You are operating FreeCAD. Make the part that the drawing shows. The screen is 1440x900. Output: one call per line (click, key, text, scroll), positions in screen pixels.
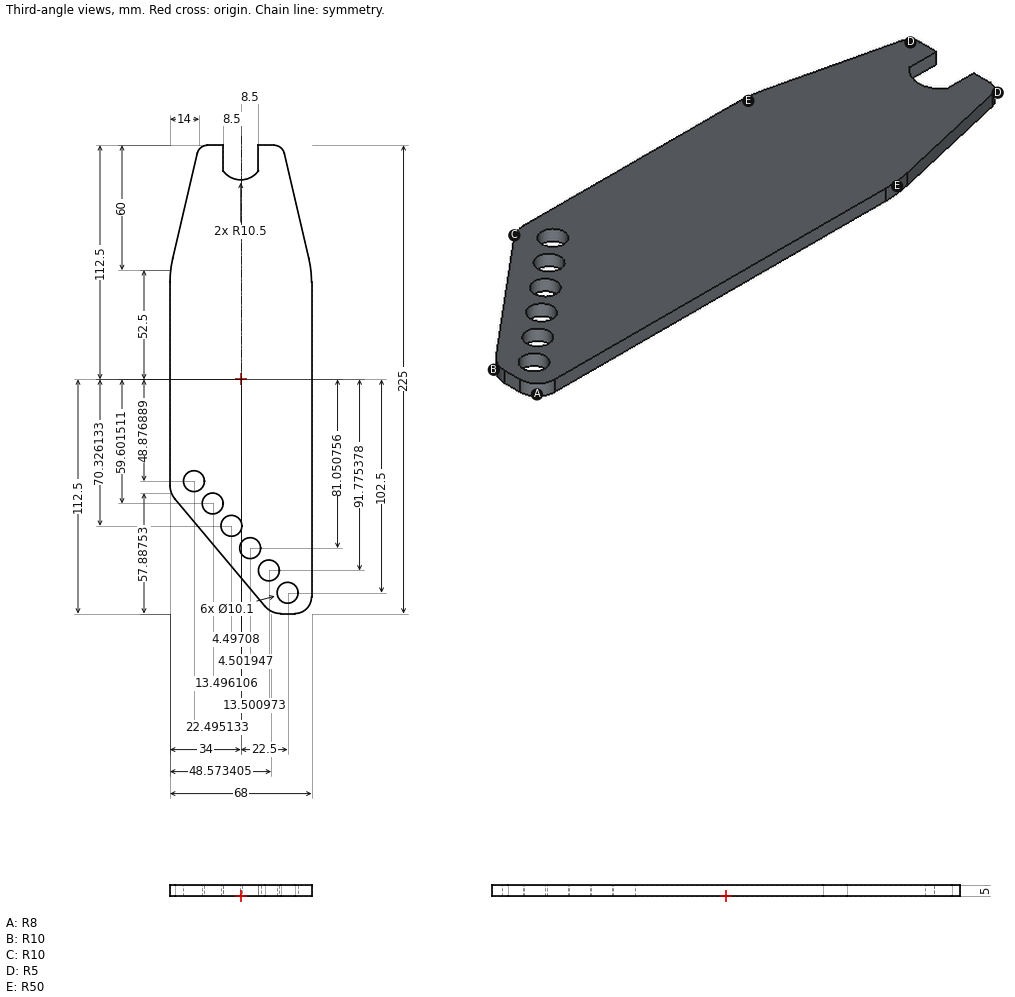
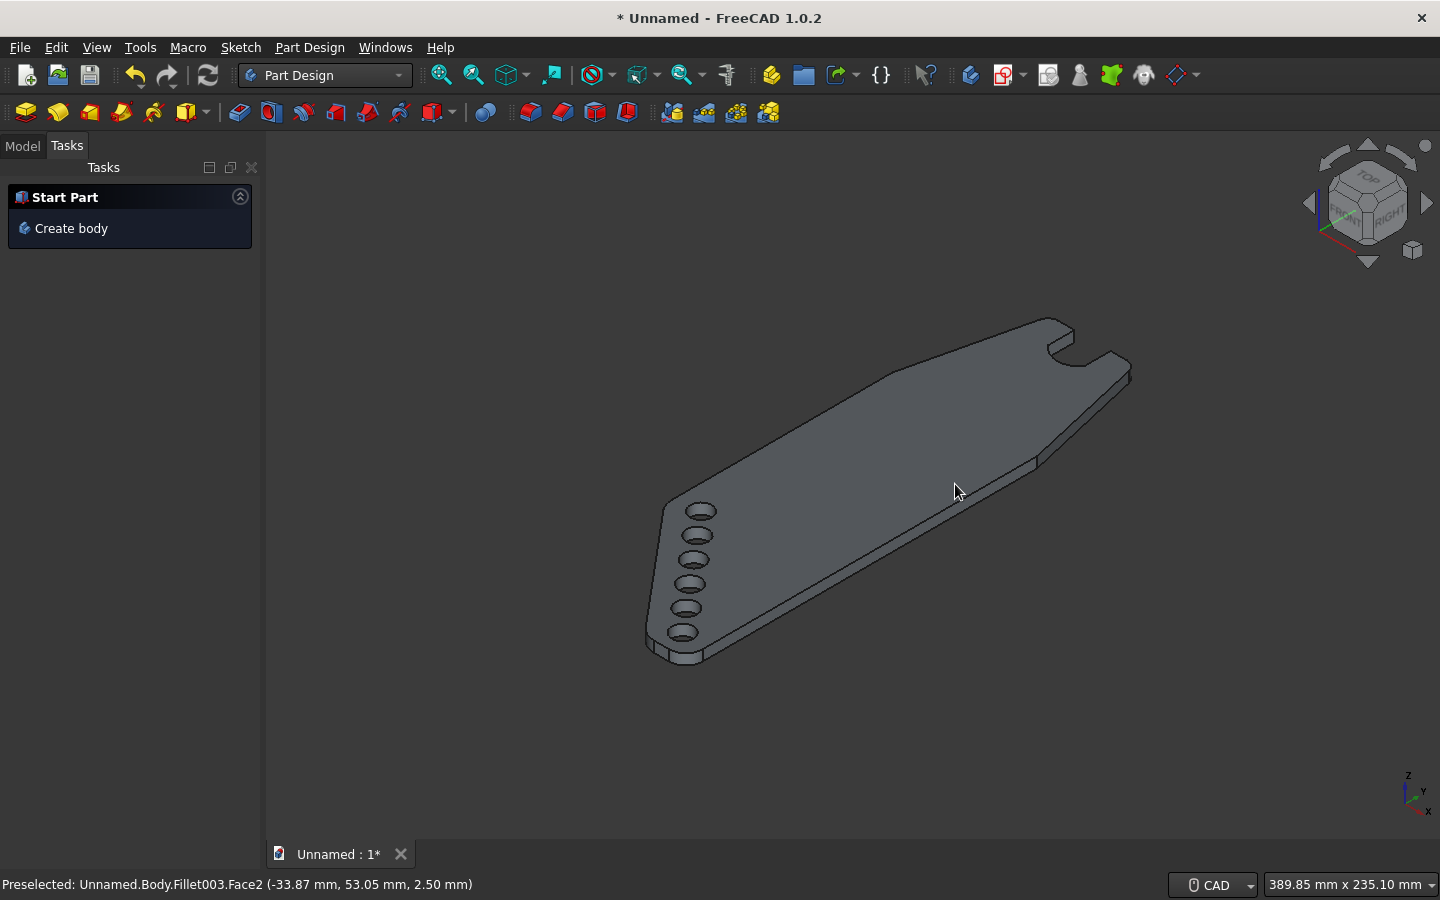
scroll(892, 378, up, 5)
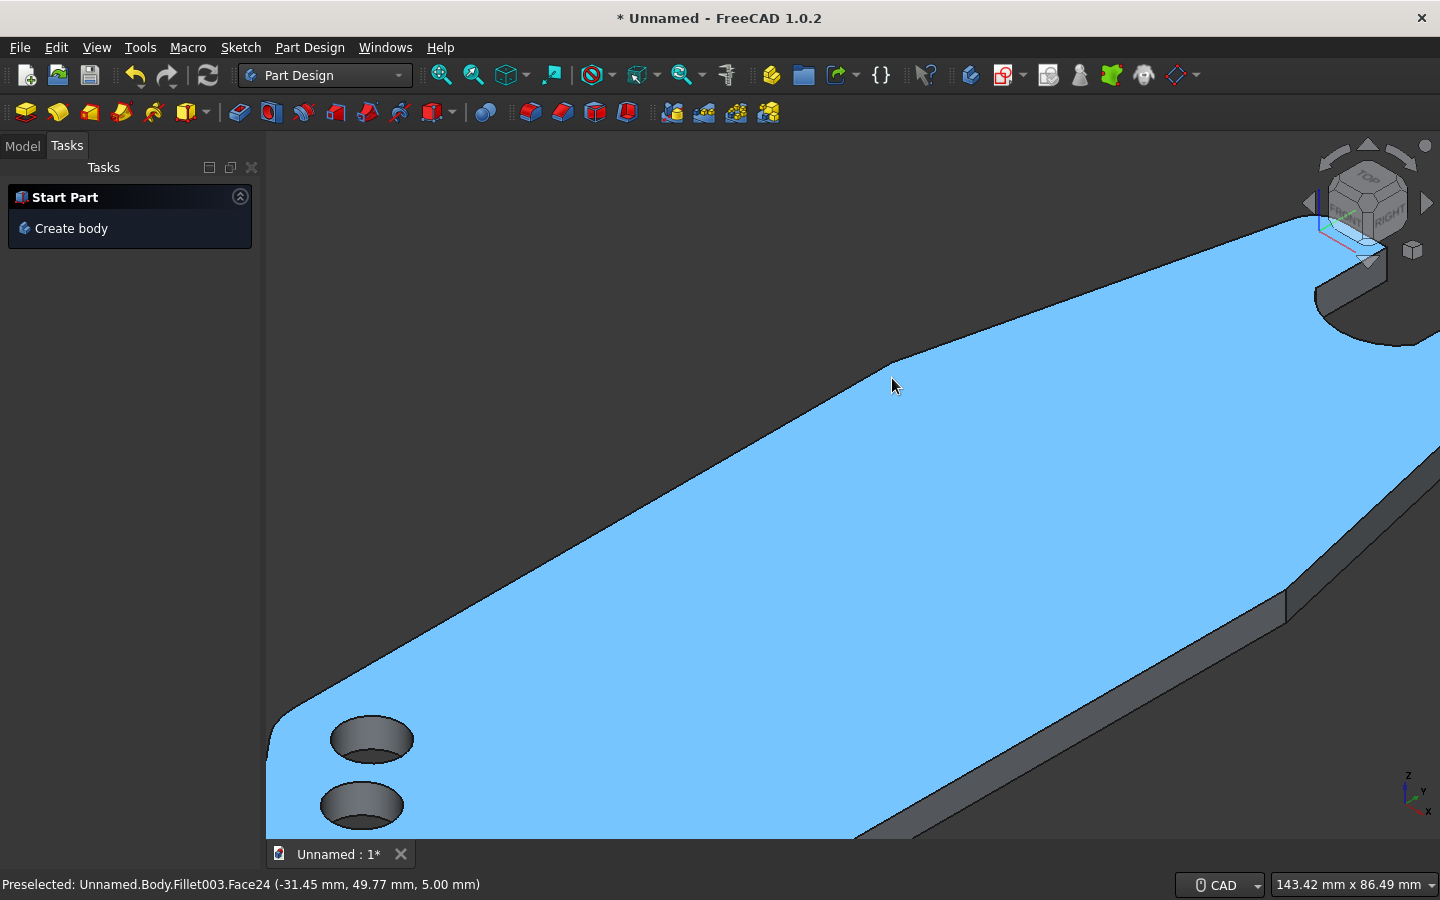
key(v)
key(f)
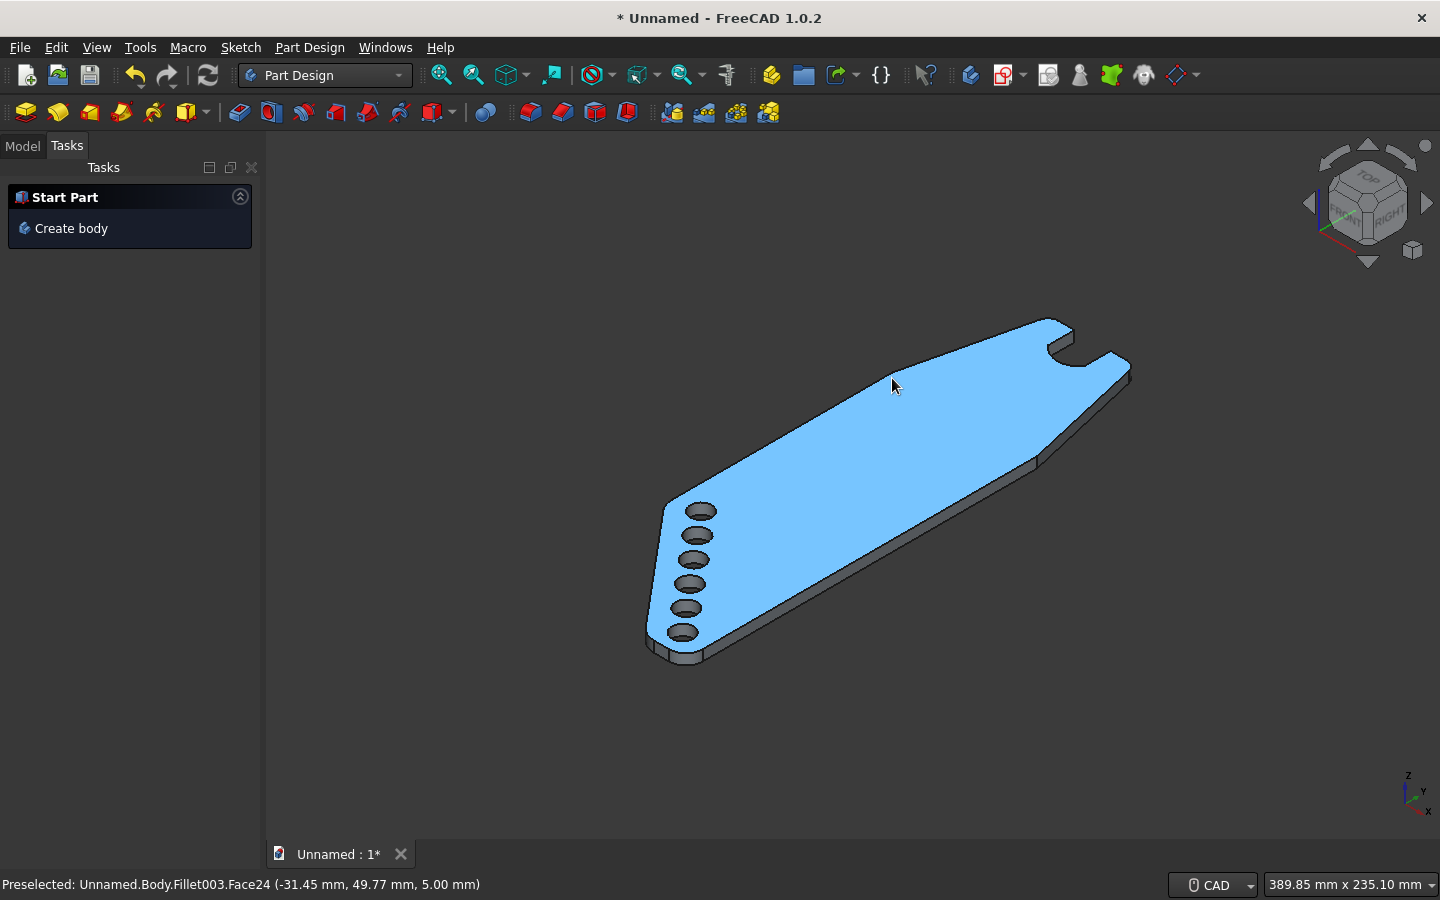
key(2)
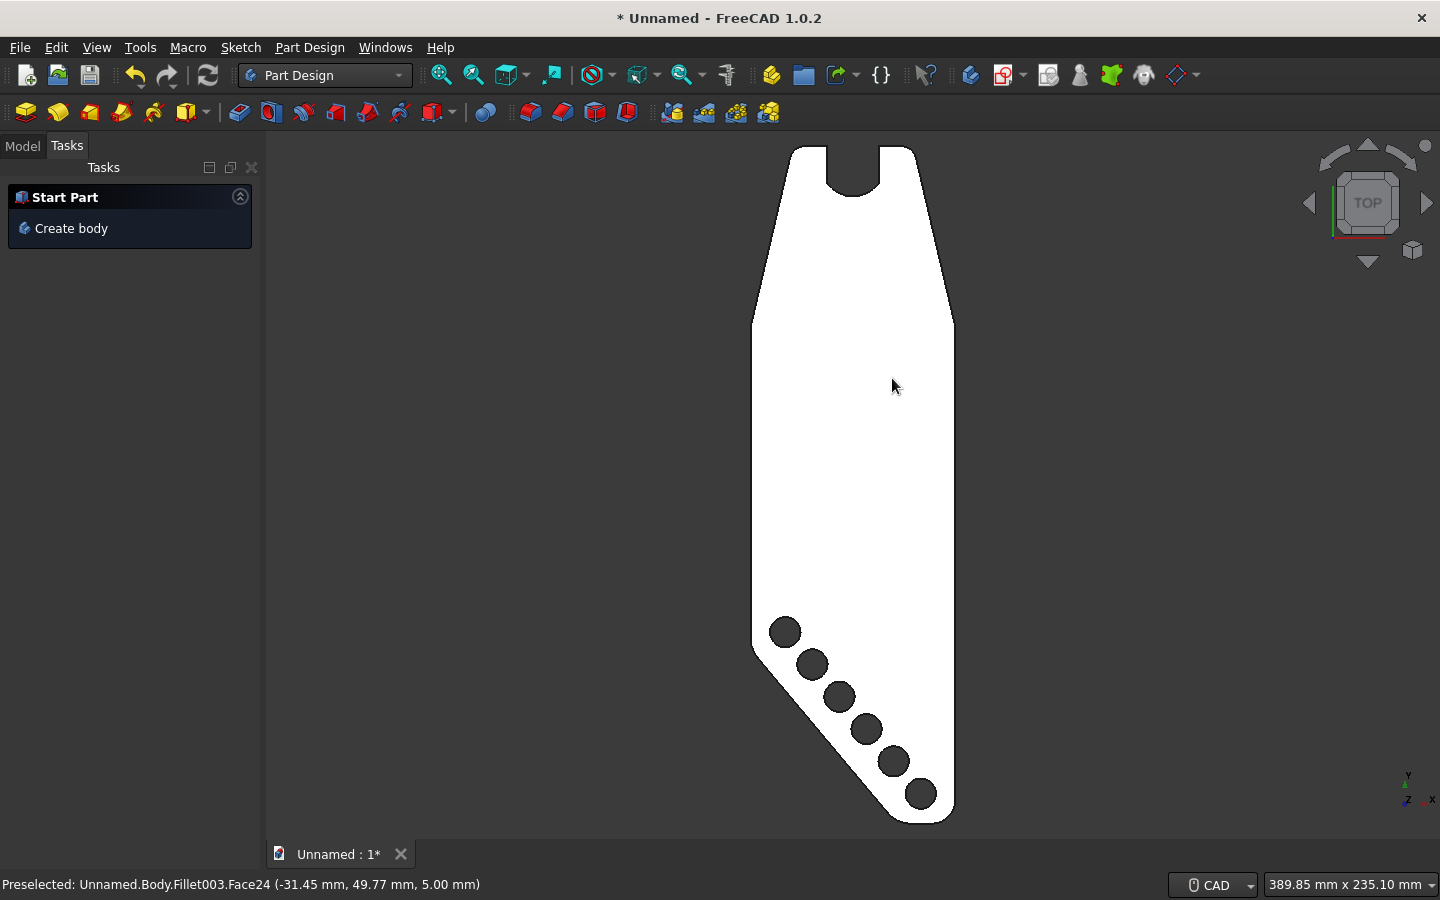
scroll(751, 326, up, 5)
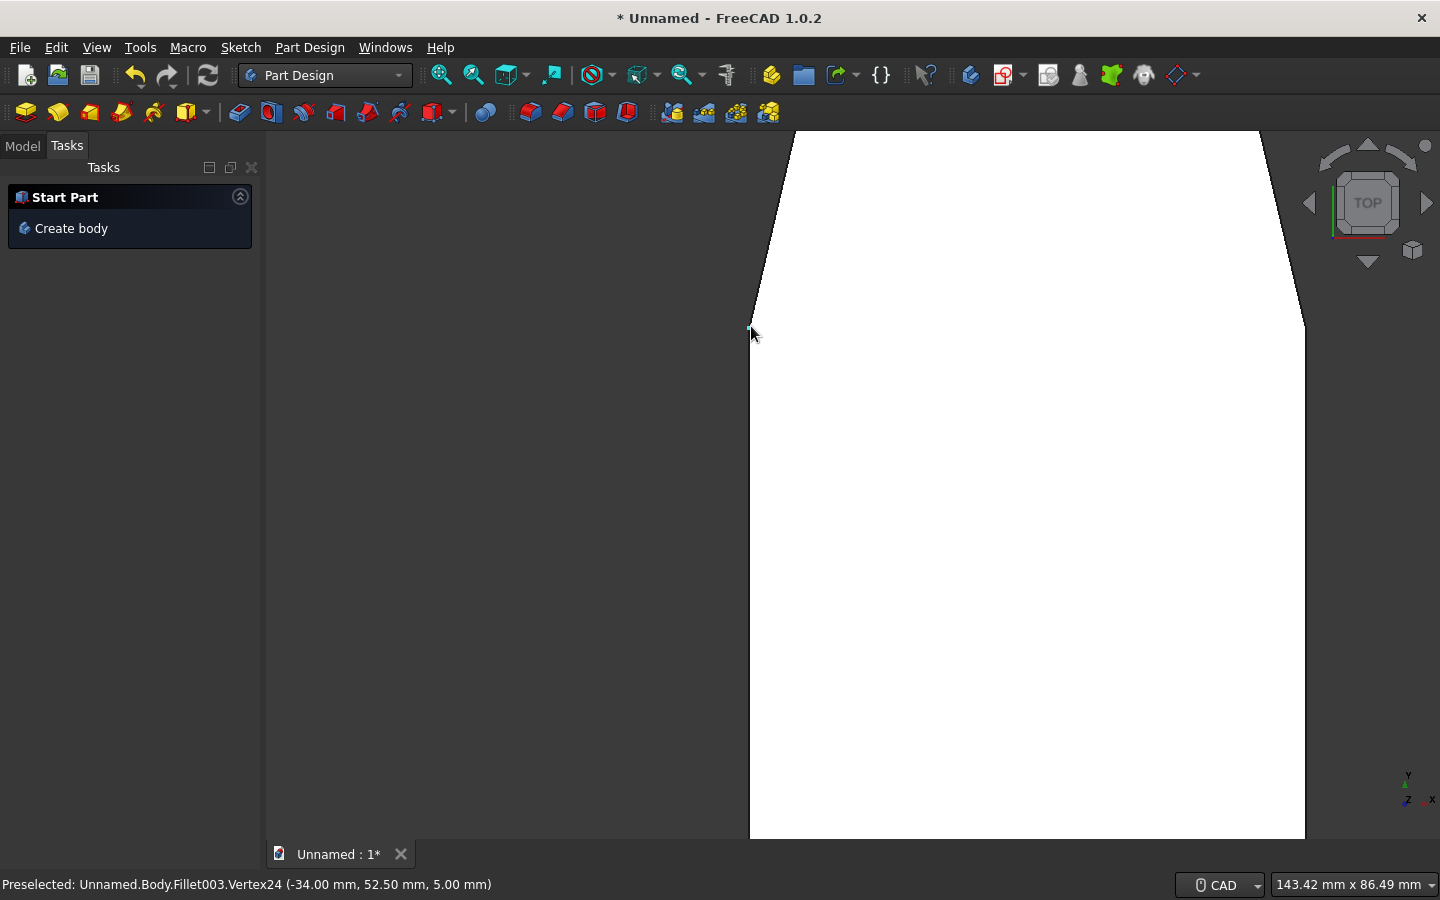
key(v)
key(f)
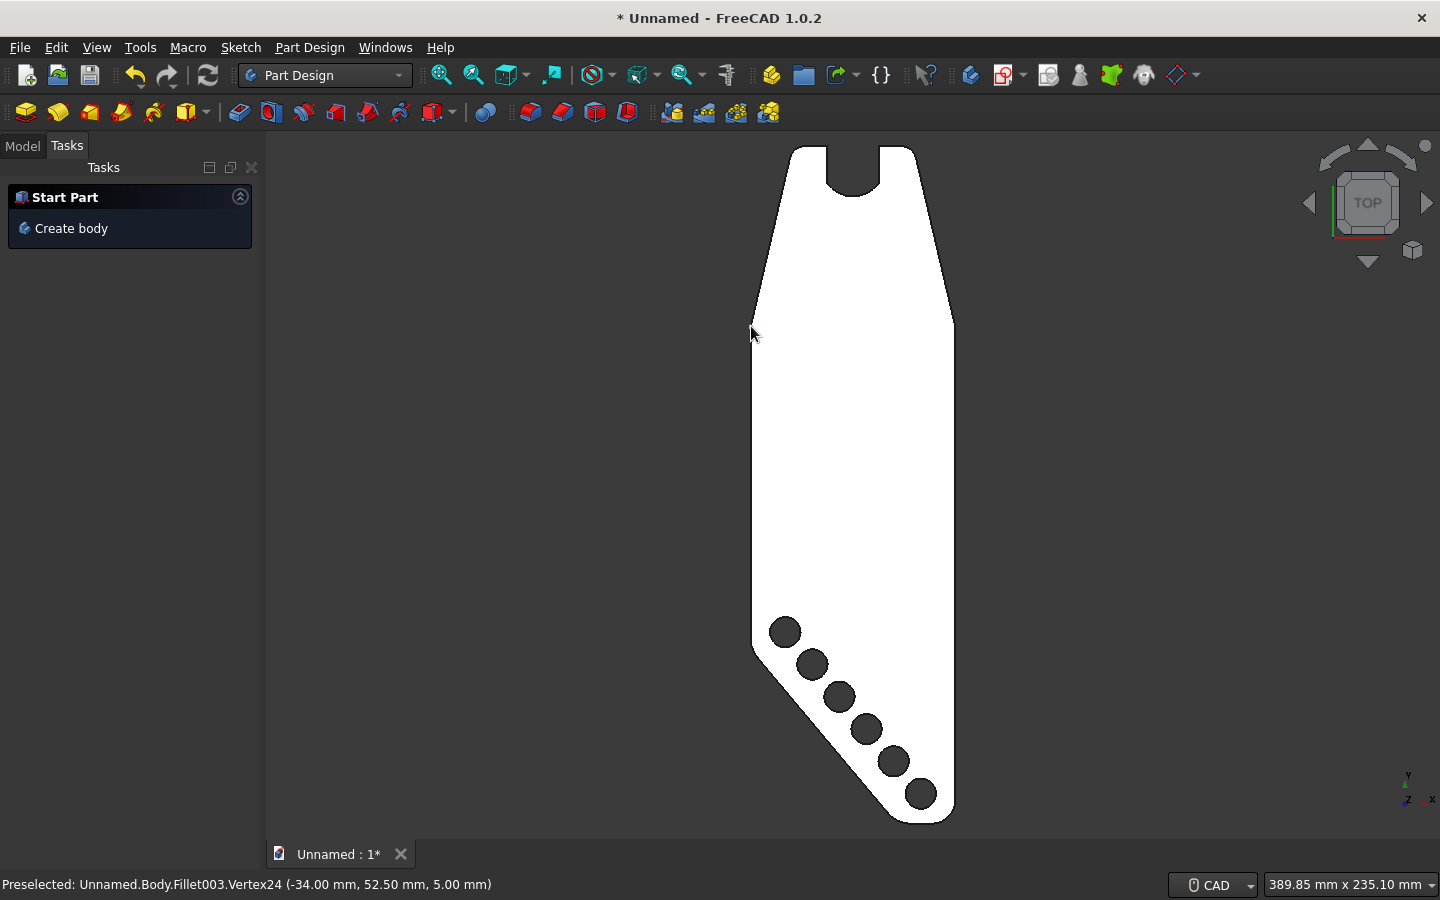
key(1)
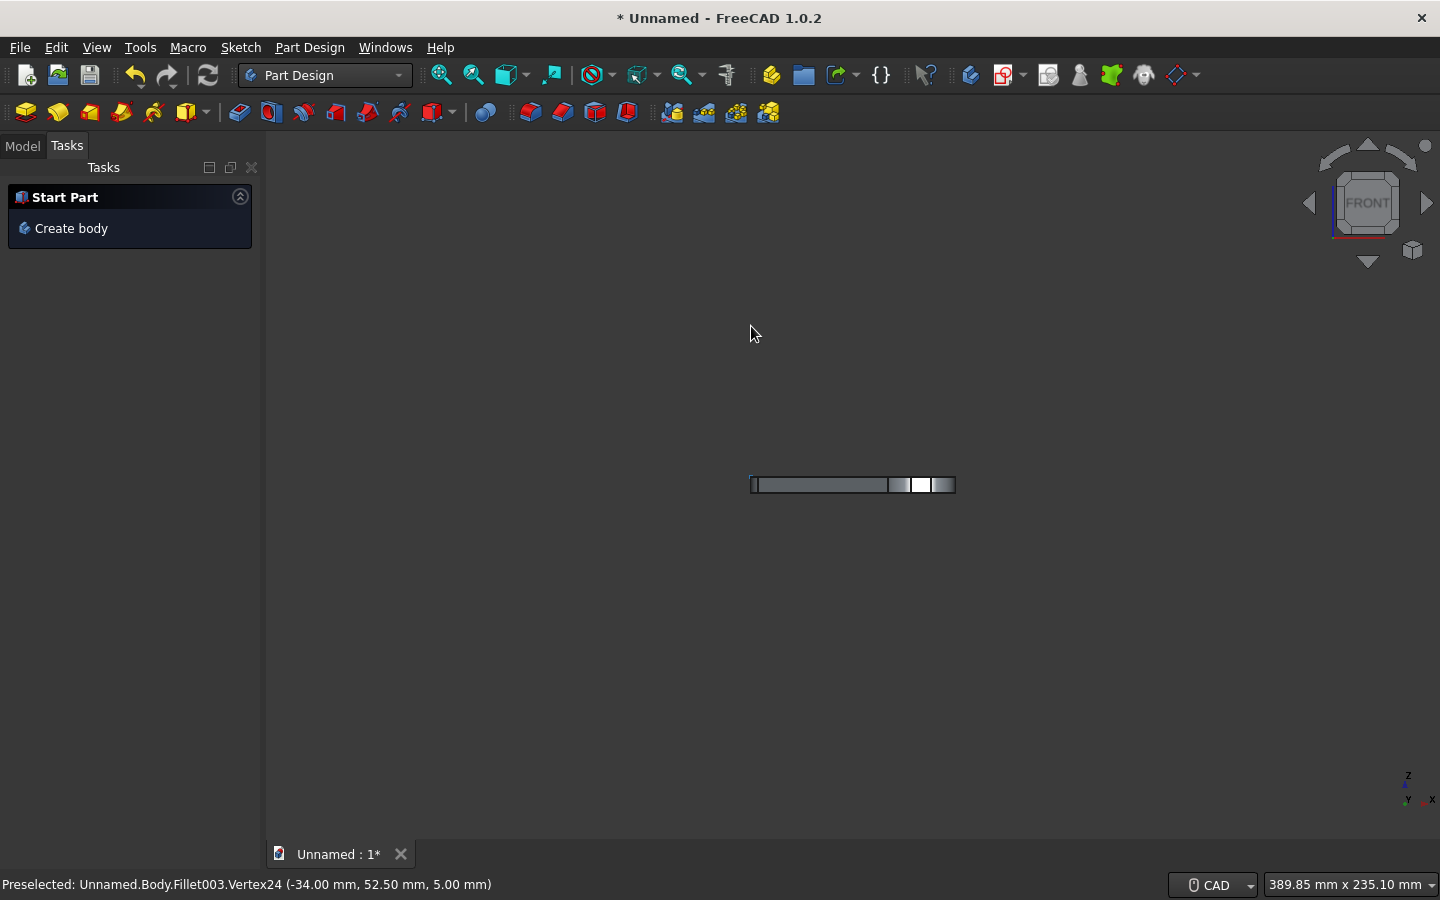
click(442, 76)